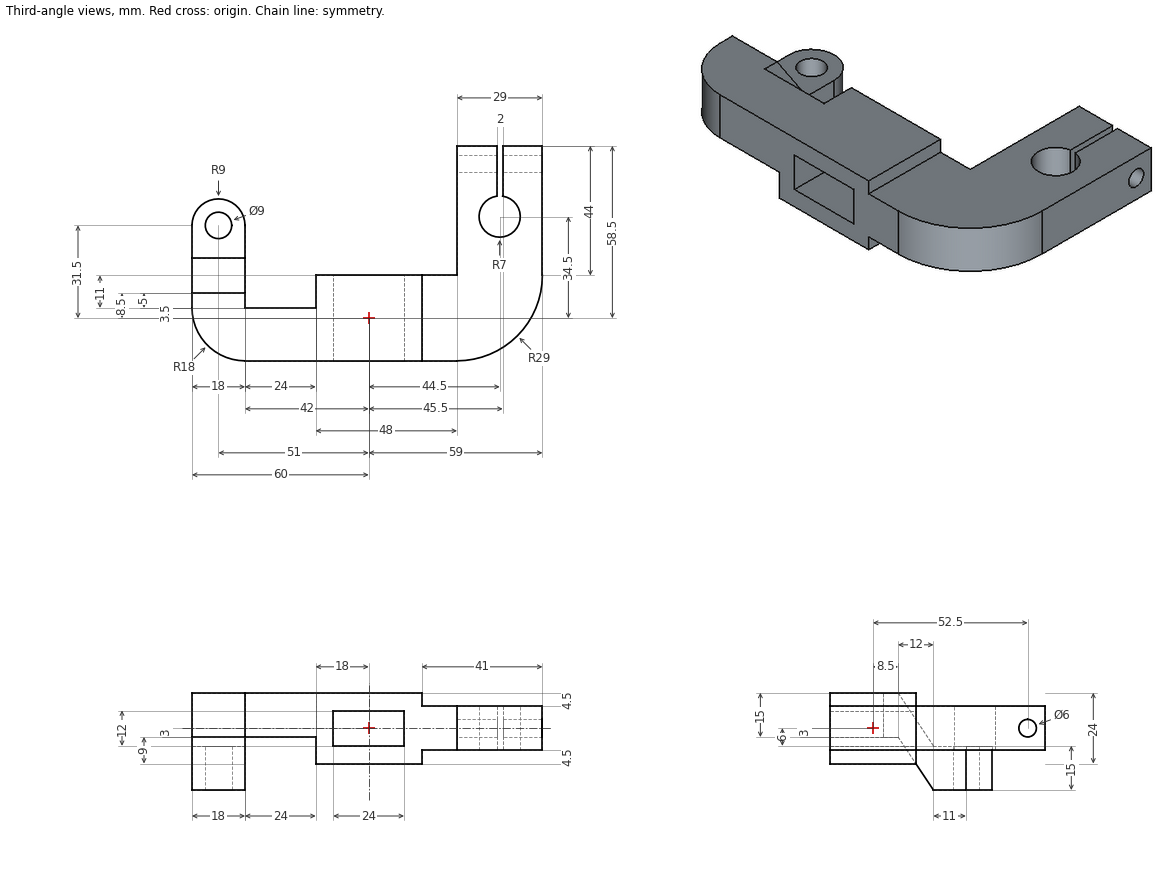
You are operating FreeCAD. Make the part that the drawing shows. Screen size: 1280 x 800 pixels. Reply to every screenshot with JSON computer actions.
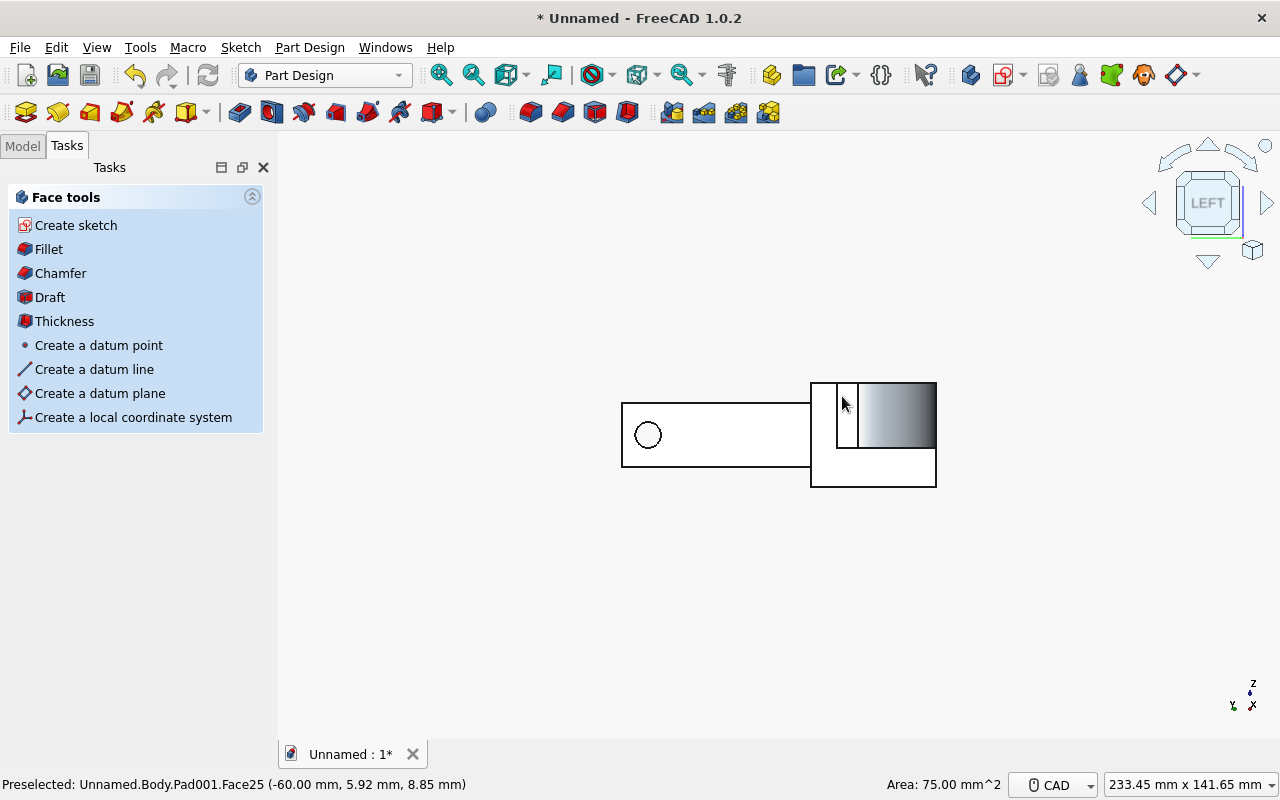
{"action": "left_click", "coordinate": [1004, 76]}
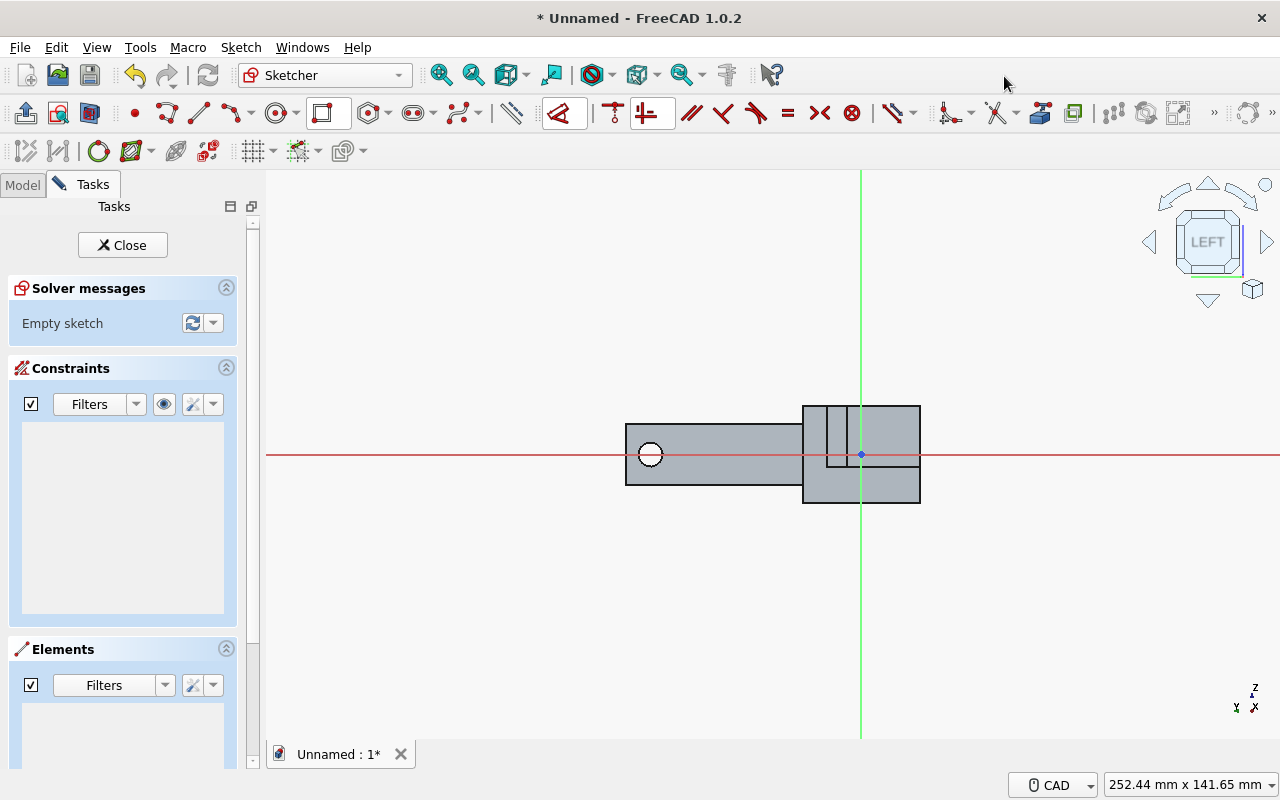
{"action": "scroll", "coordinate": [853, 483], "scroll_direction": "up", "scroll_amount": 5}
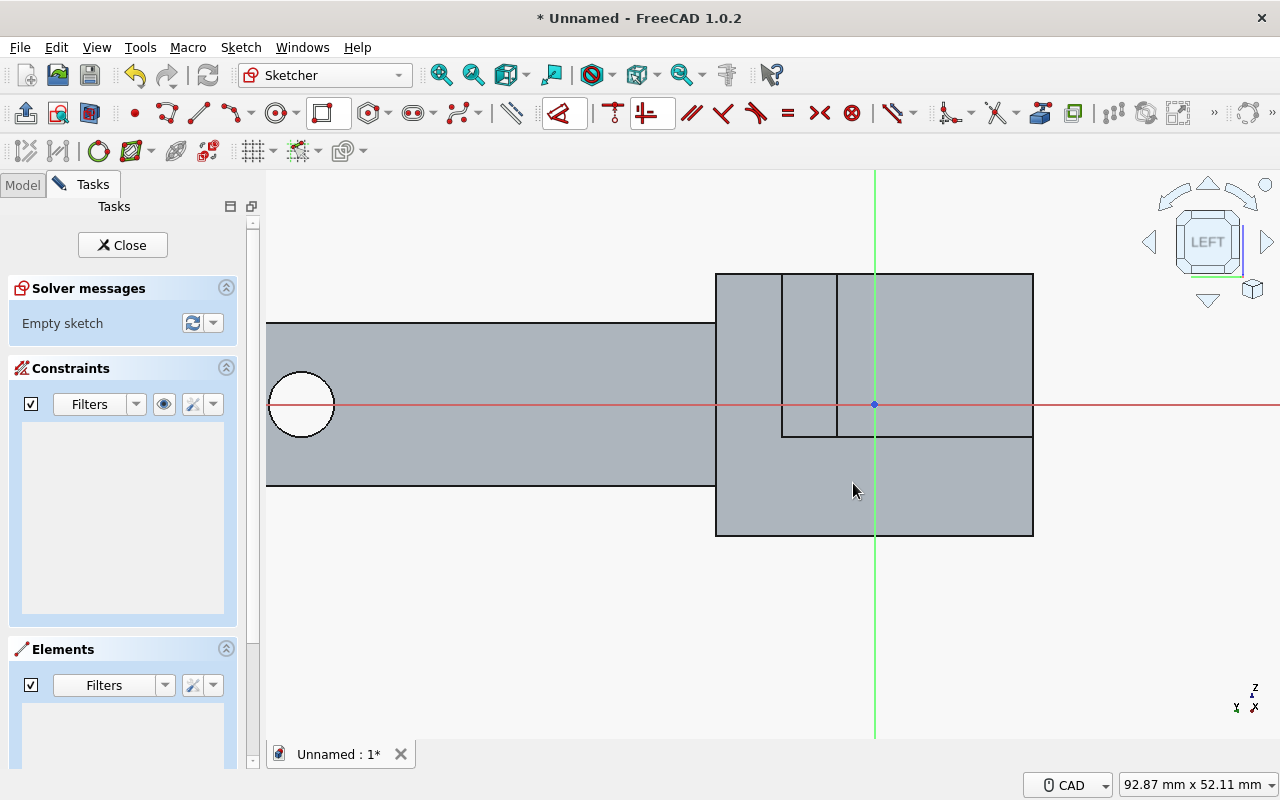
{"action": "left_click", "coordinate": [168, 114]}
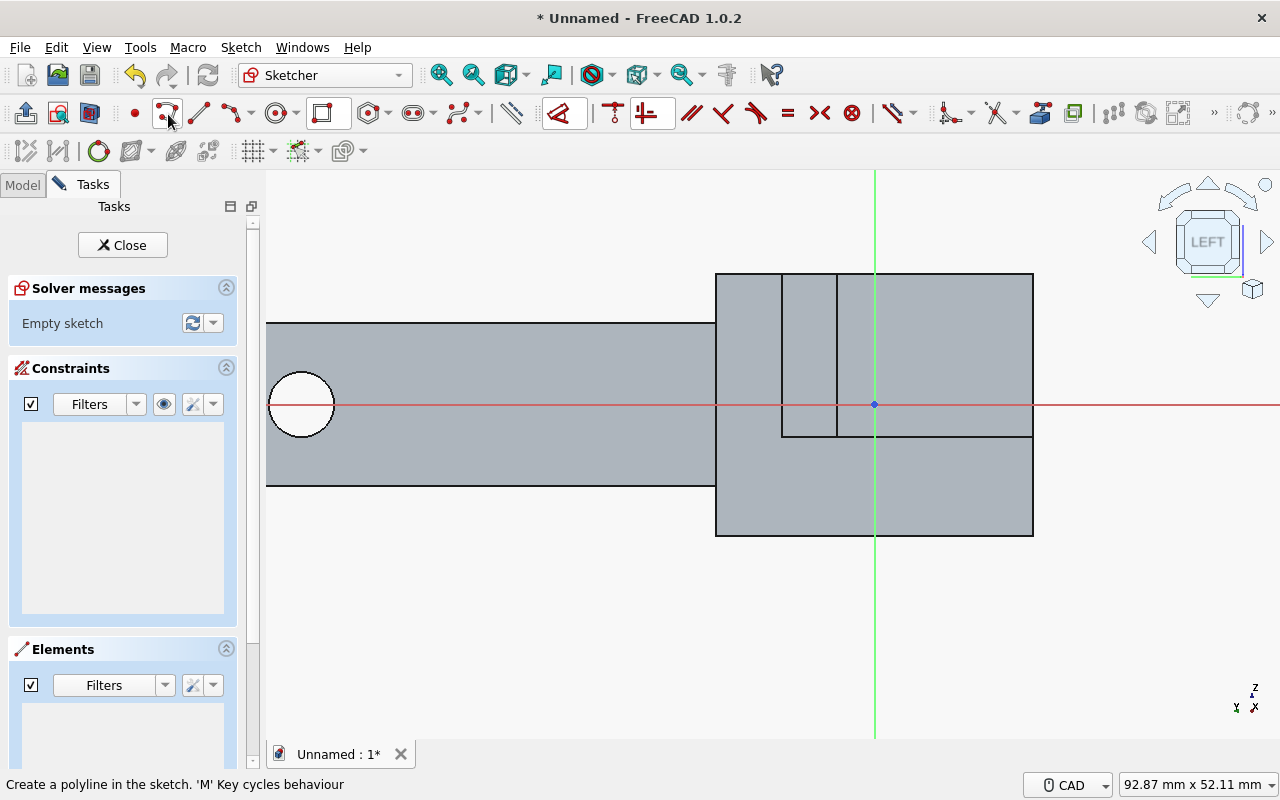
{"action": "left_click", "coordinate": [782, 437]}
{"action": "left_click", "coordinate": [782, 274]}
{"action": "left_click", "coordinate": [651, 470]}
{"action": "left_click", "coordinate": [531, 470]}
{"action": "left_click", "coordinate": [531, 634]}
{"action": "left_click", "coordinate": [651, 634]}
{"action": "left_click", "coordinate": [782, 438]}
{"action": "key", "text": "Escape"}
{"action": "key", "text": "Escape"}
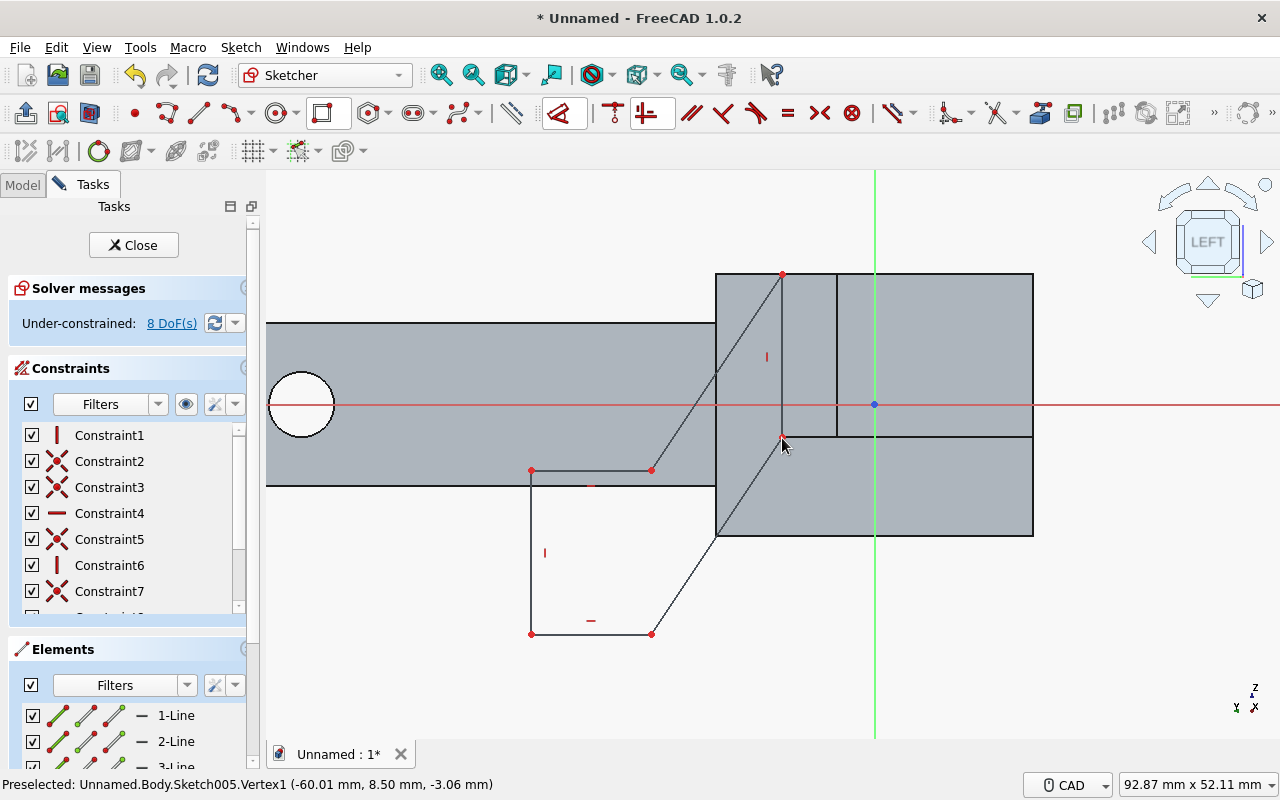
{"action": "left_click", "coordinate": [782, 389]}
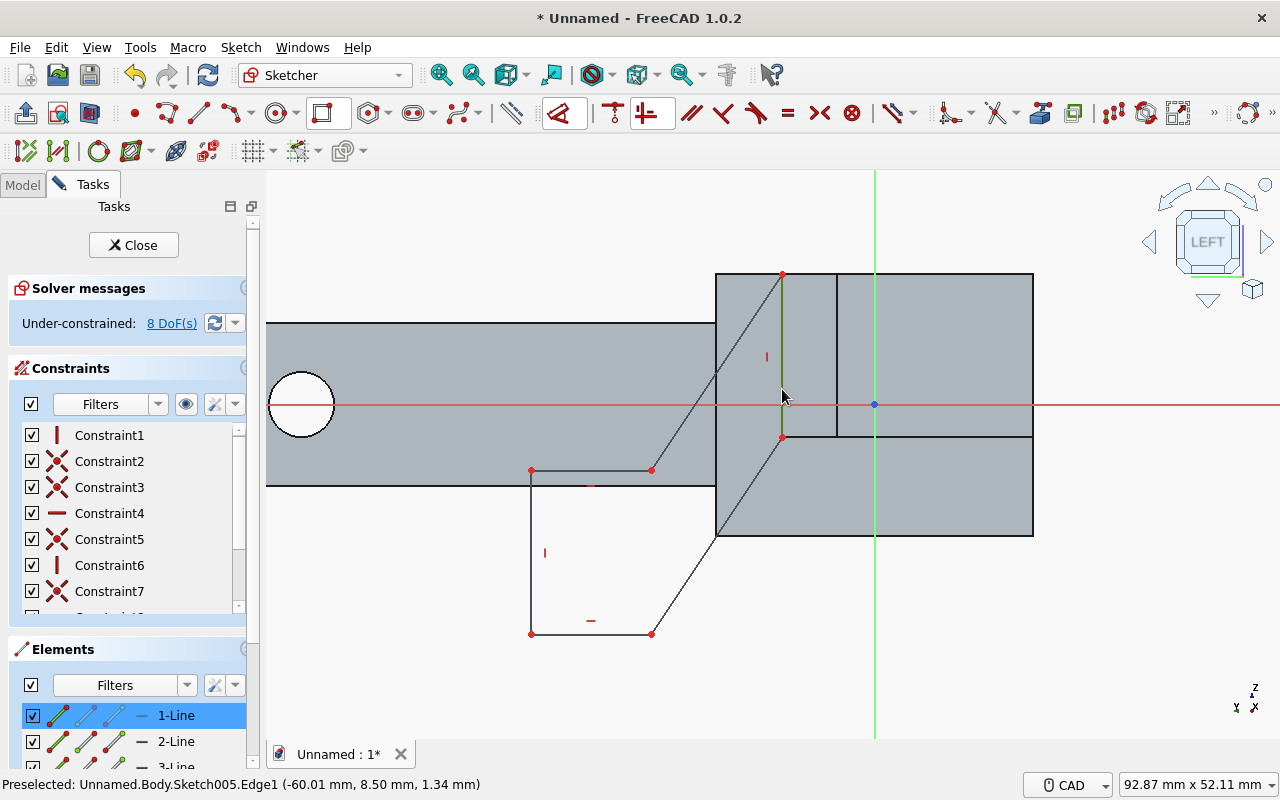
{"action": "left_click", "coordinate": [582, 114]}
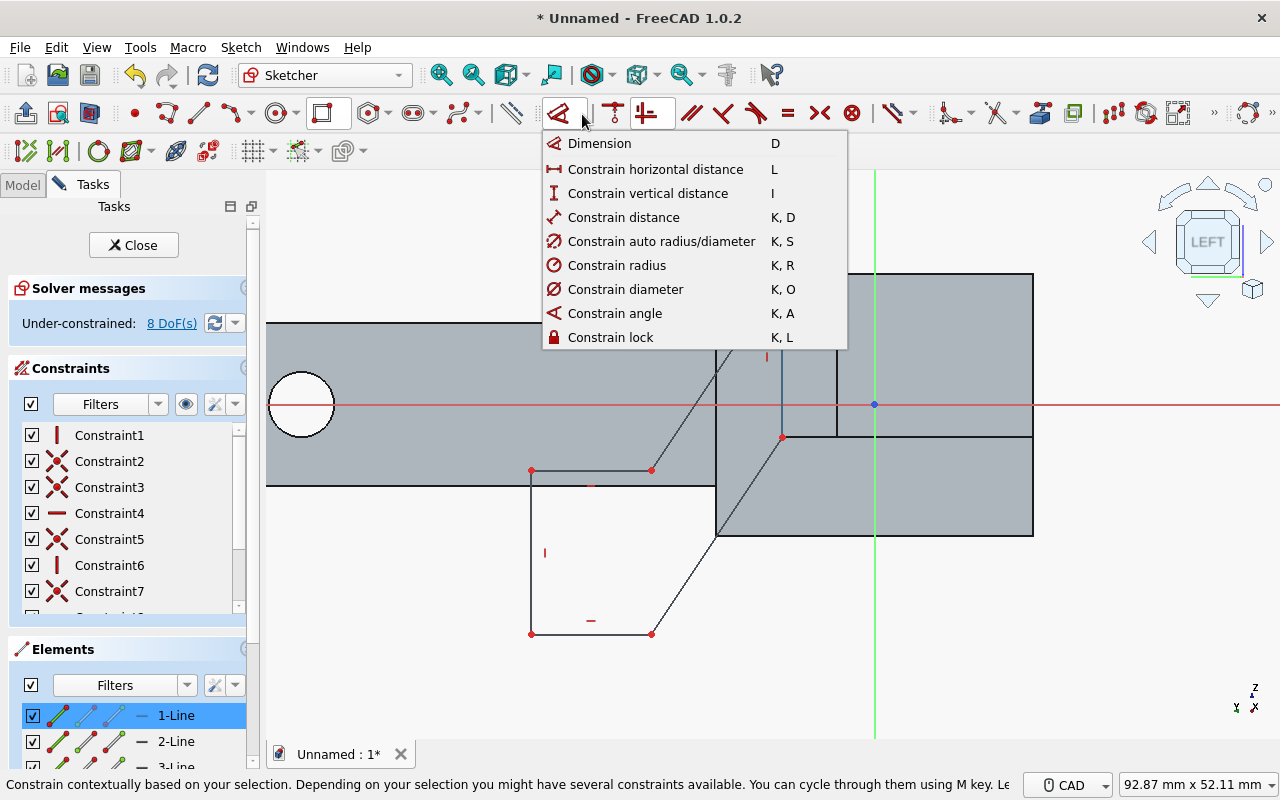
{"action": "left_click", "coordinate": [695, 193]}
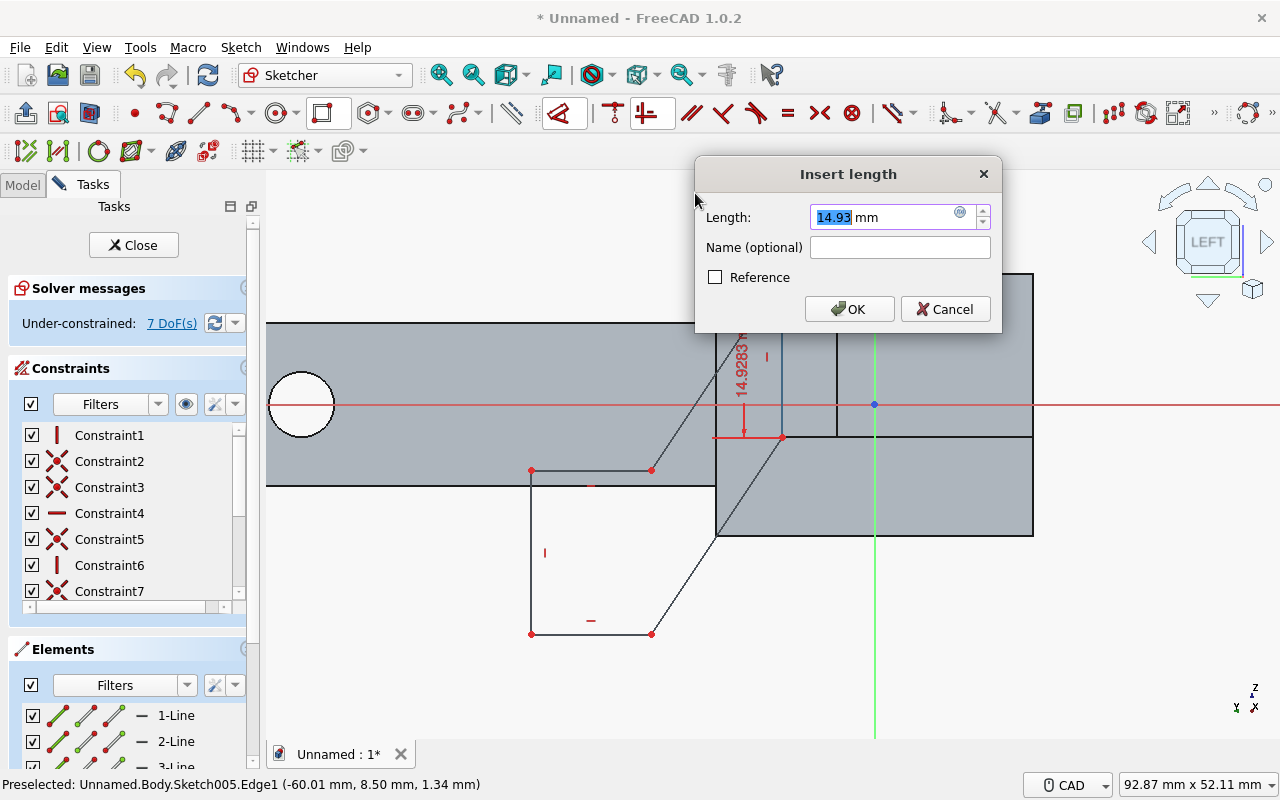
{"action": "type", "text": "15"}
{"action": "key", "text": "Return"}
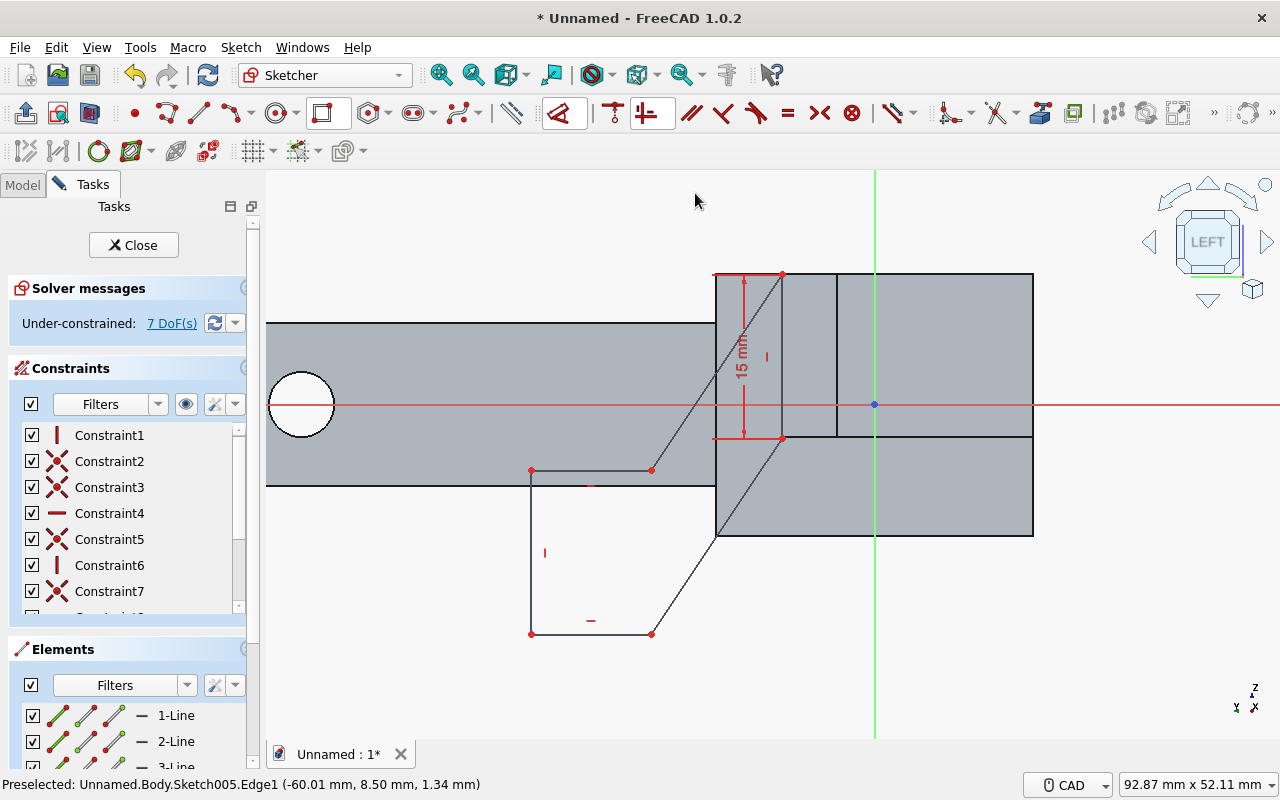
{"action": "left_click", "coordinate": [615, 471]}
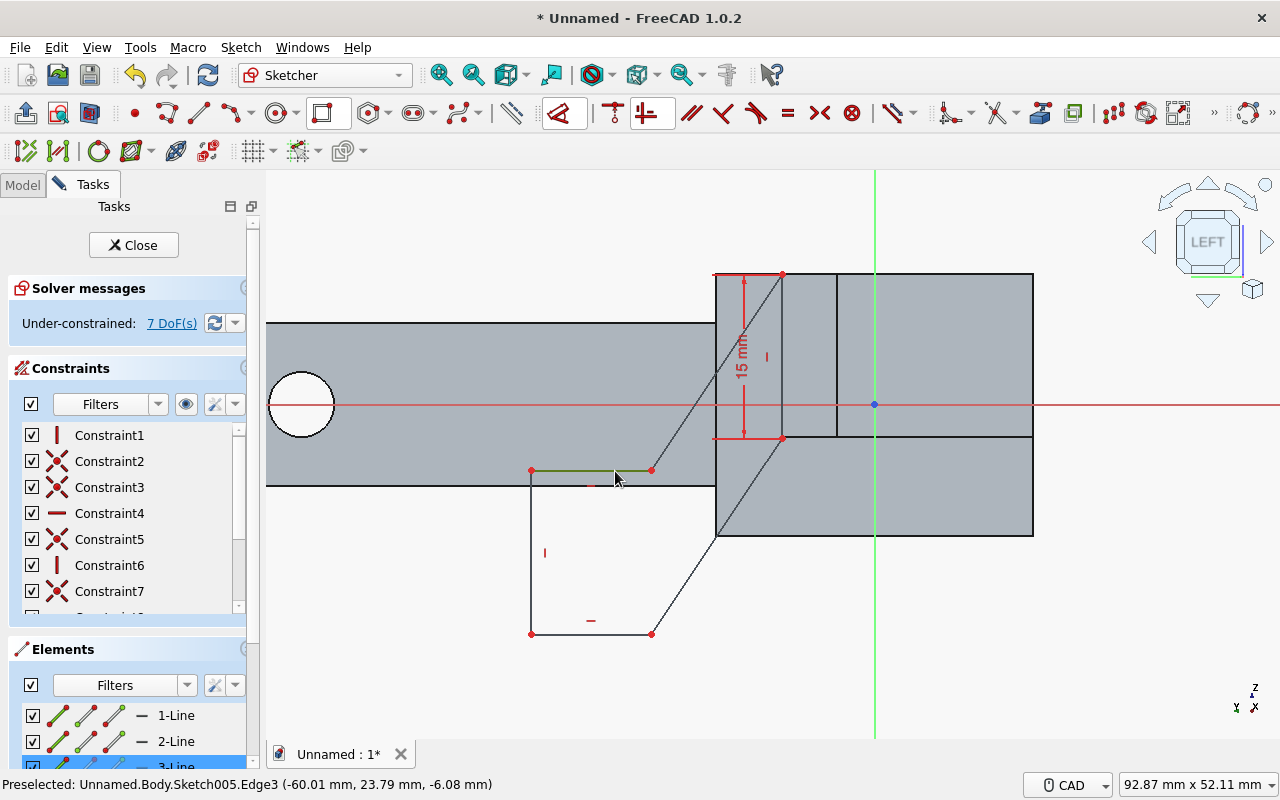
{"action": "left_click", "coordinate": [582, 114]}